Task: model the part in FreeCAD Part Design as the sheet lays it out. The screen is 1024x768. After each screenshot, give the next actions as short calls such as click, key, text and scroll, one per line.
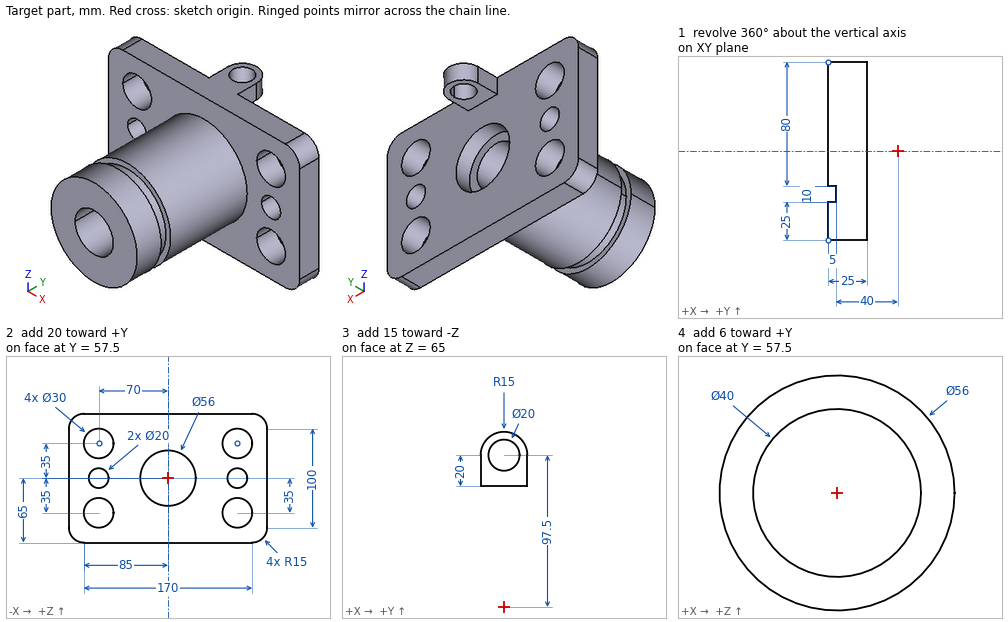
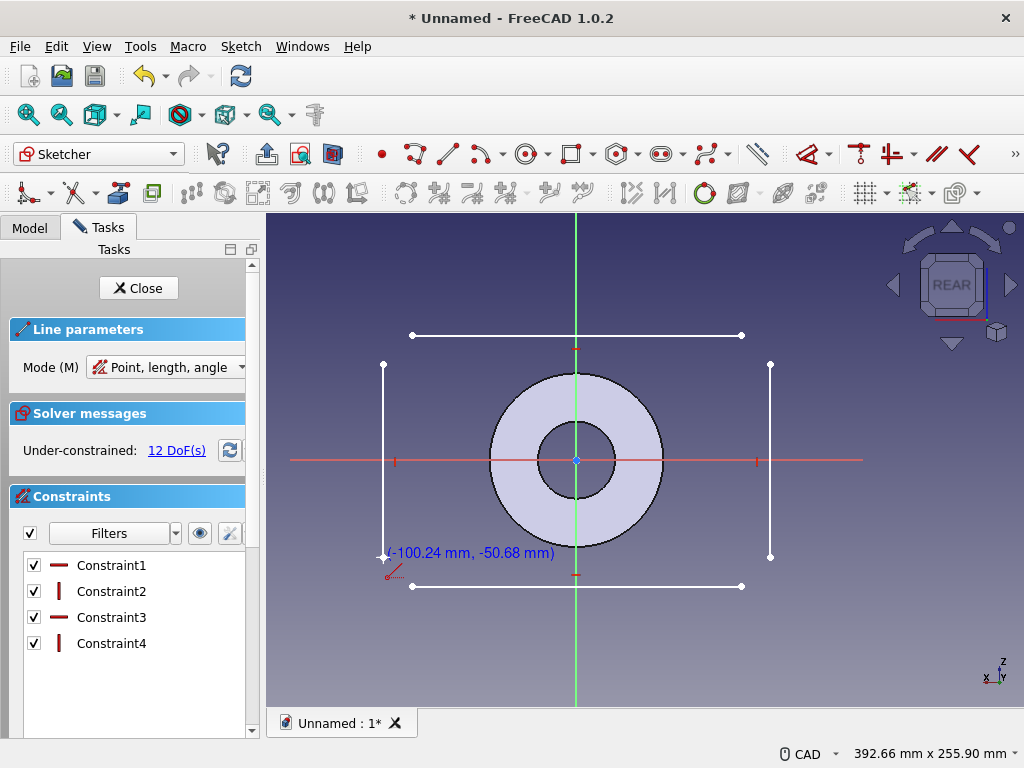
click(502, 154)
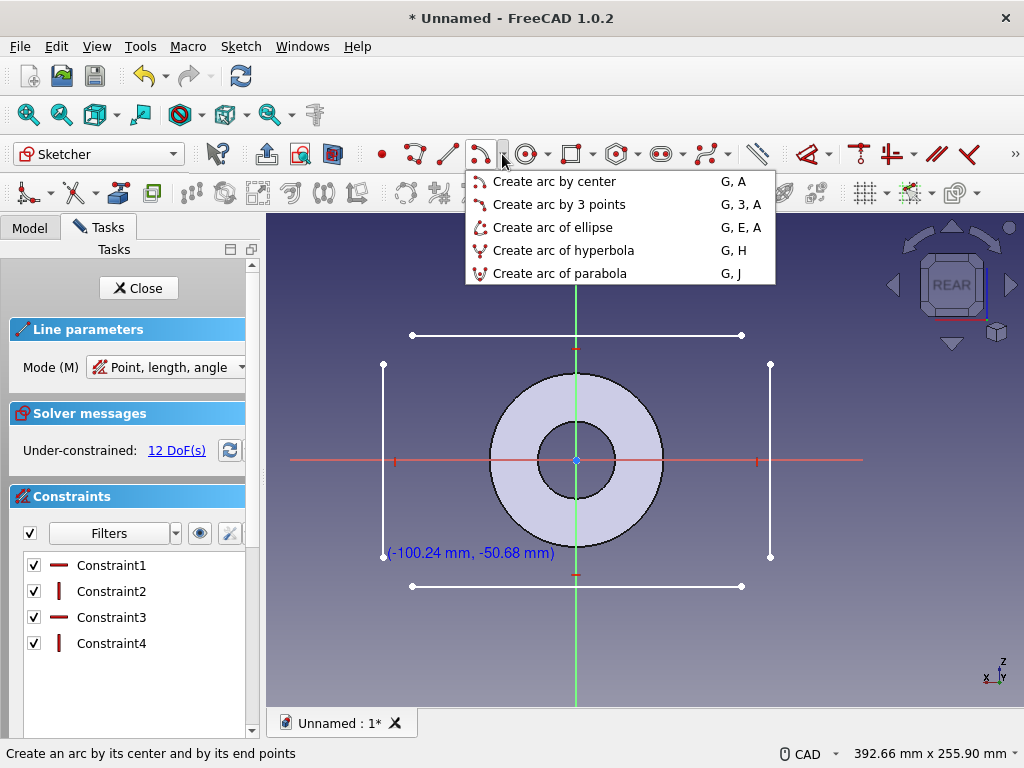
click(620, 204)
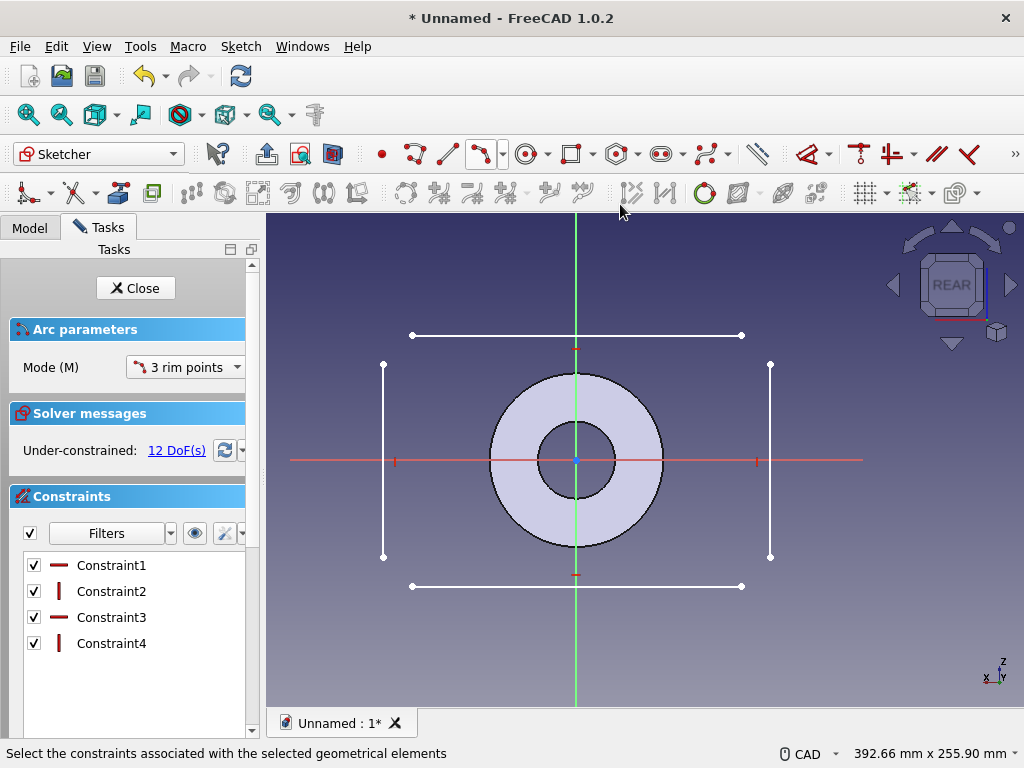
click(741, 587)
click(770, 558)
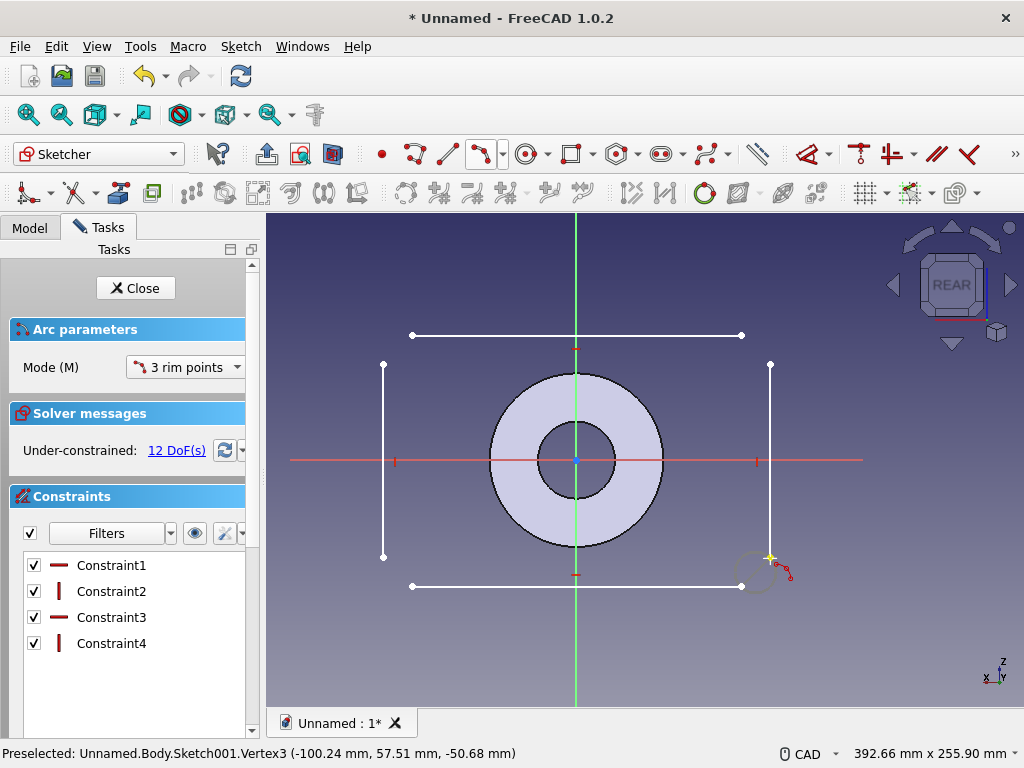
scroll(761, 577, up, 4)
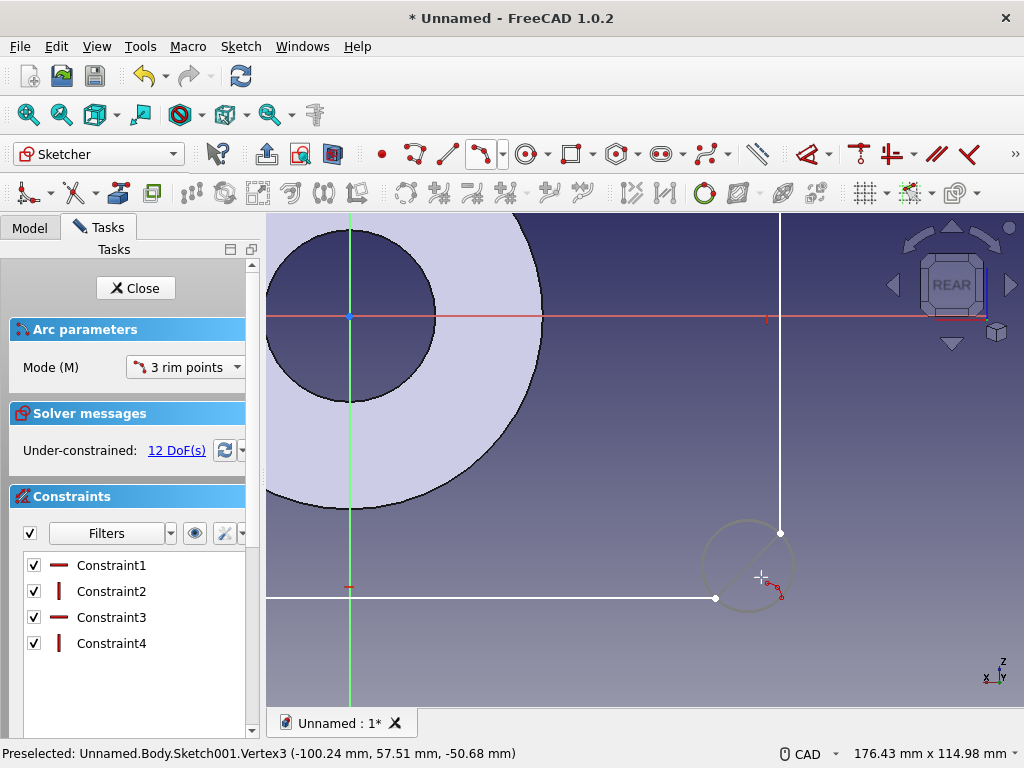
click(760, 576)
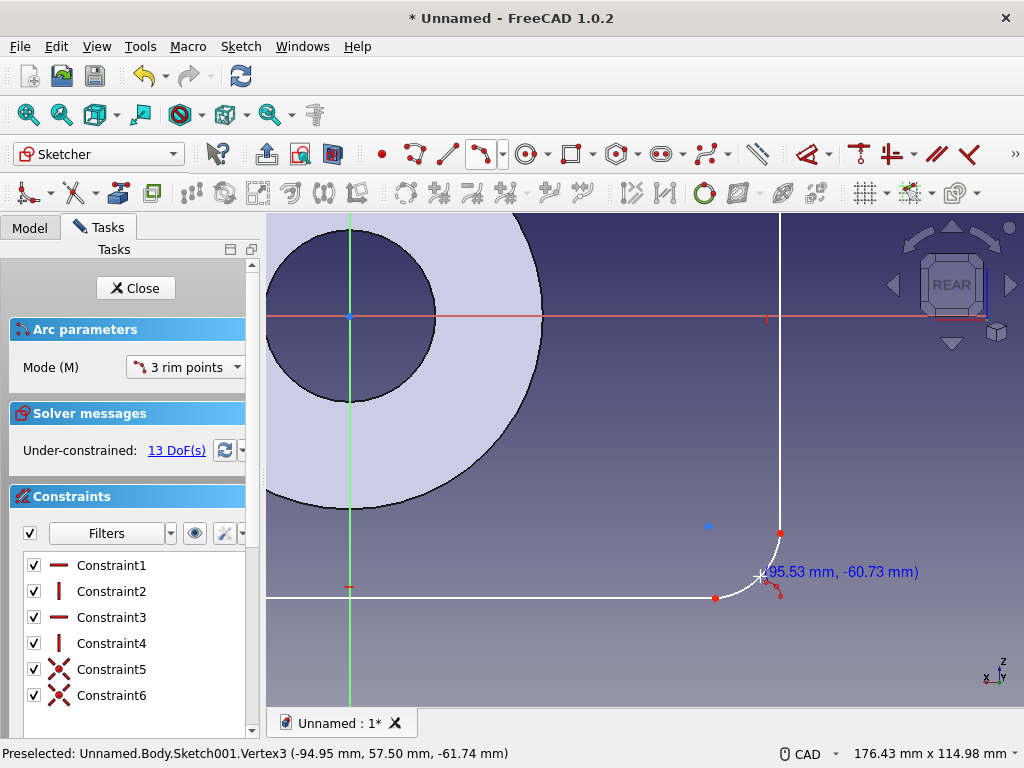
scroll(762, 577, down, 4)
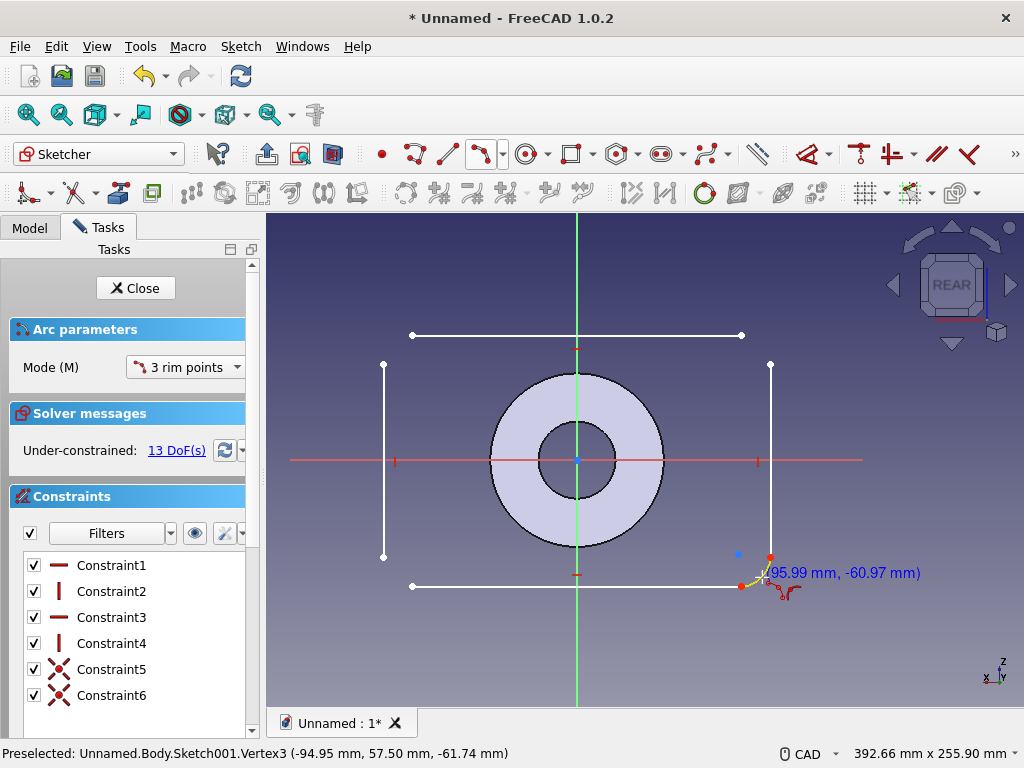
click(771, 365)
click(742, 336)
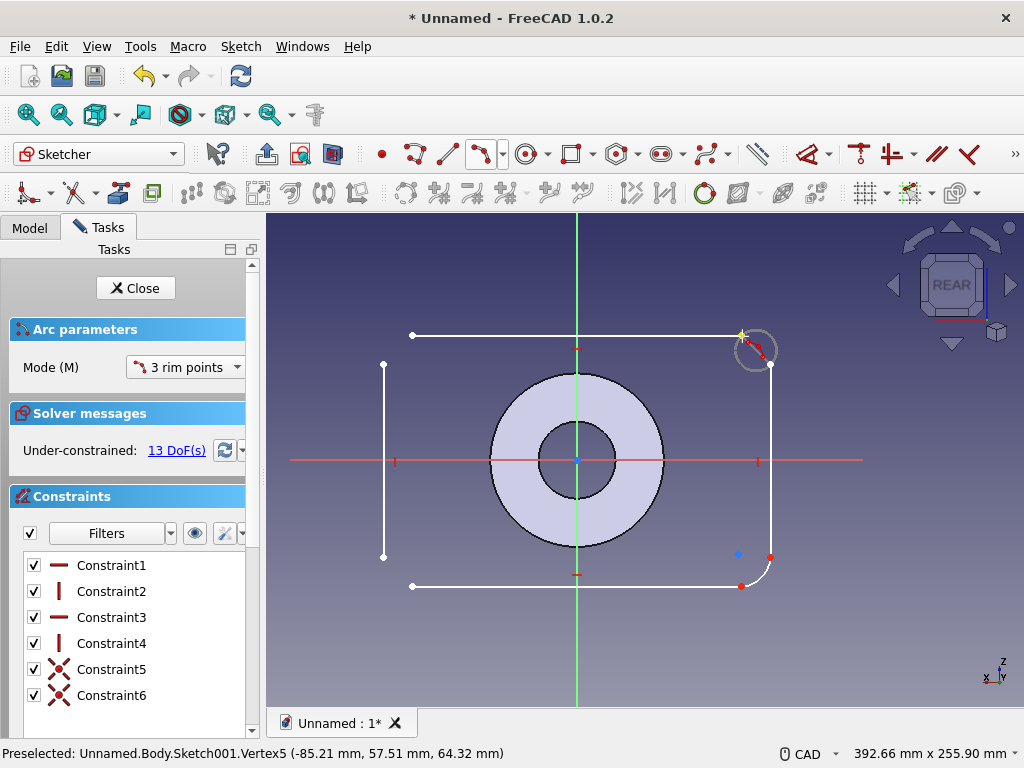
scroll(762, 343, up, 4)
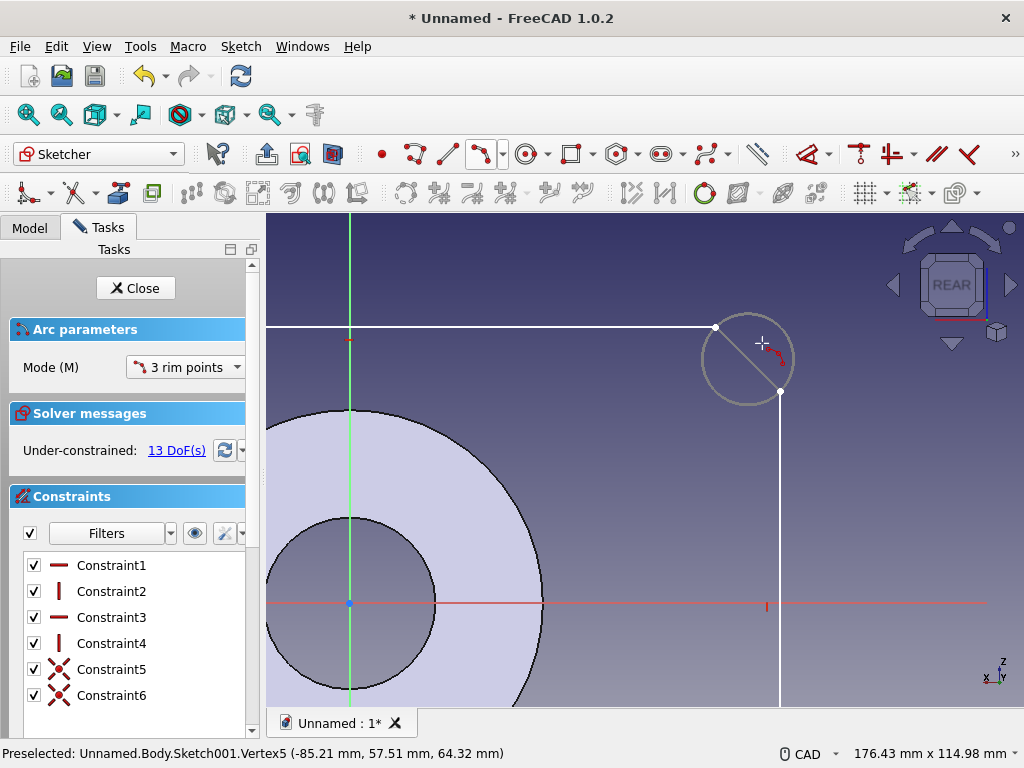
click(760, 343)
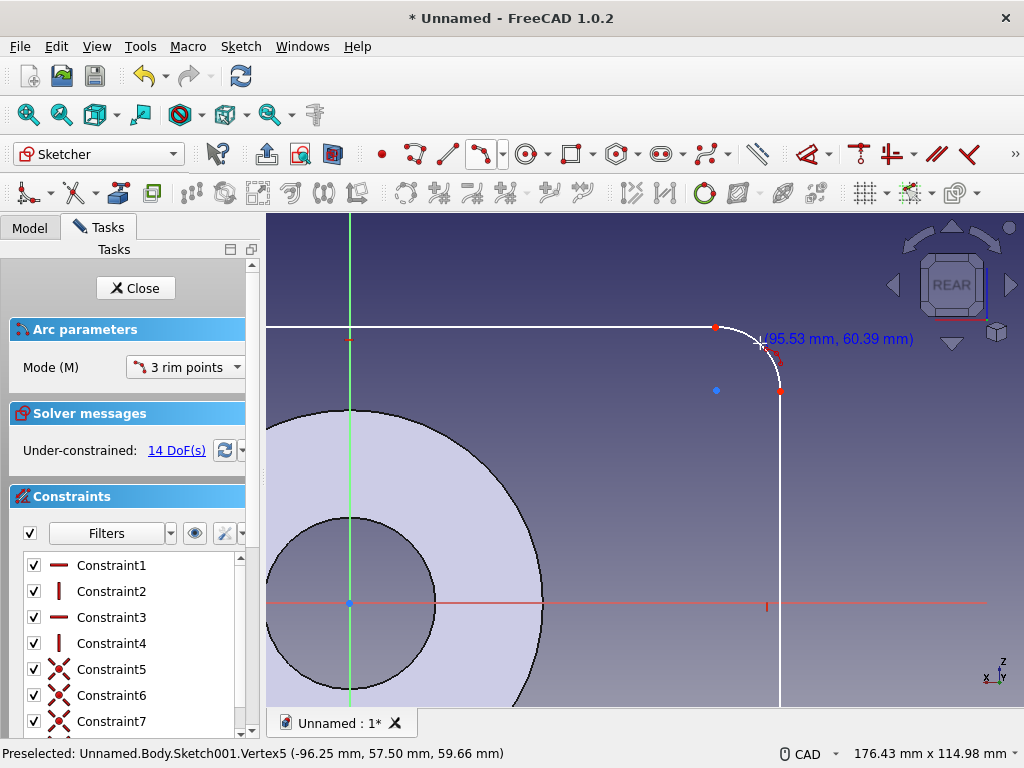
scroll(762, 343, down, 4)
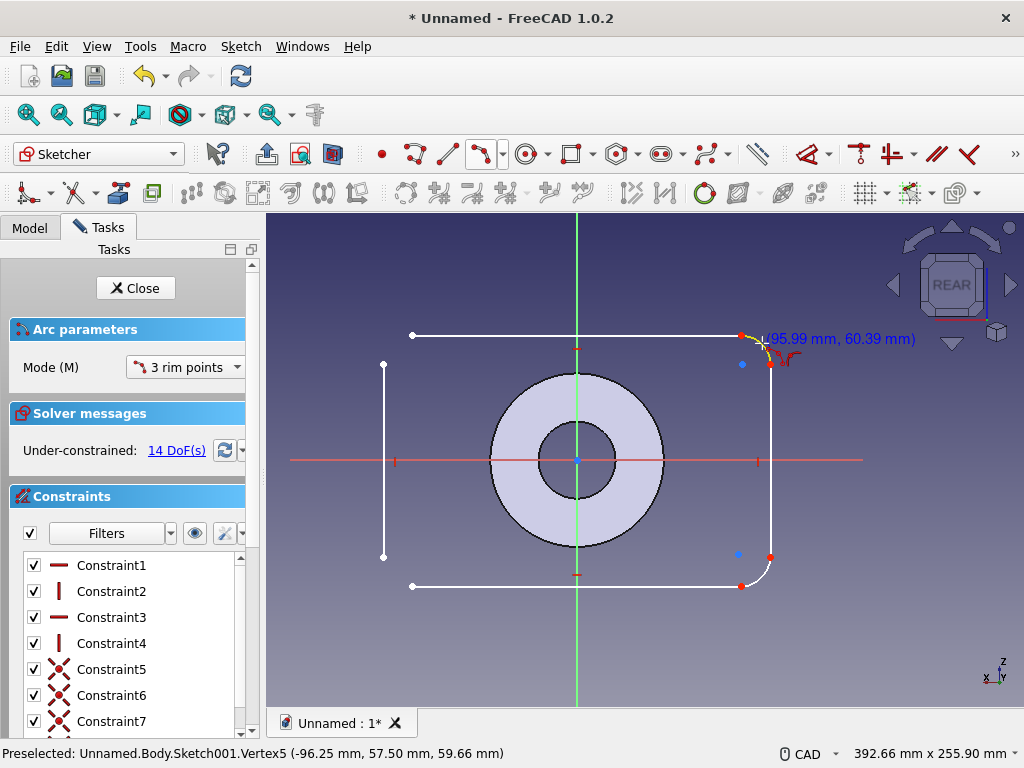
click(413, 336)
click(384, 365)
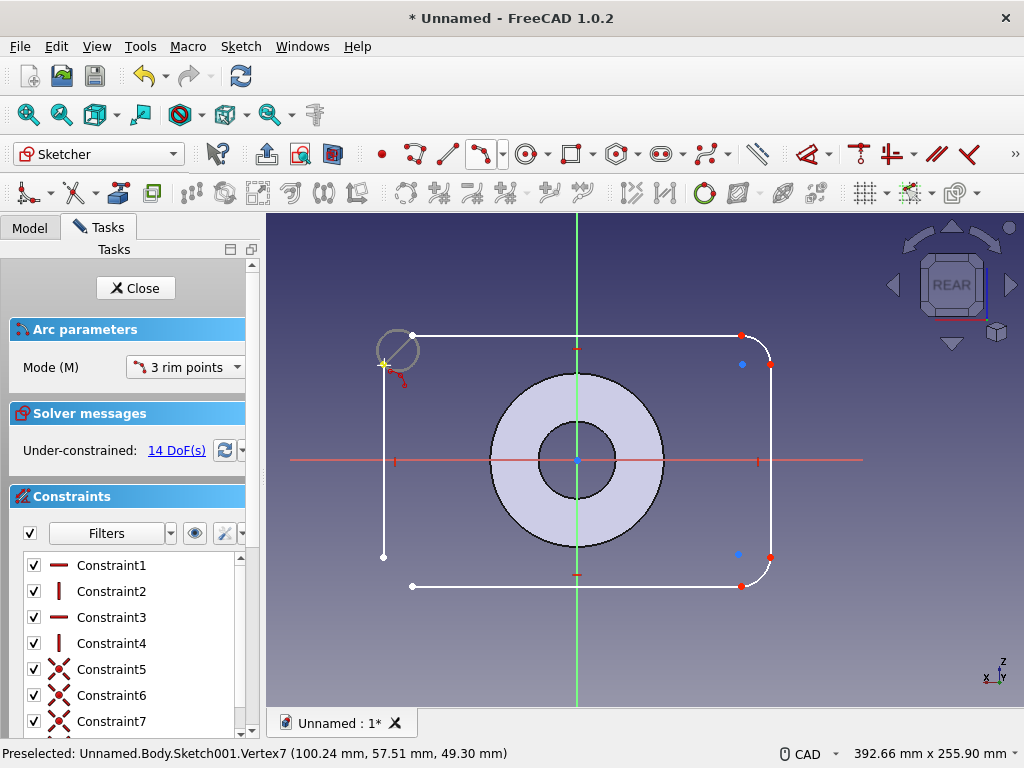
scroll(392, 343, up, 4)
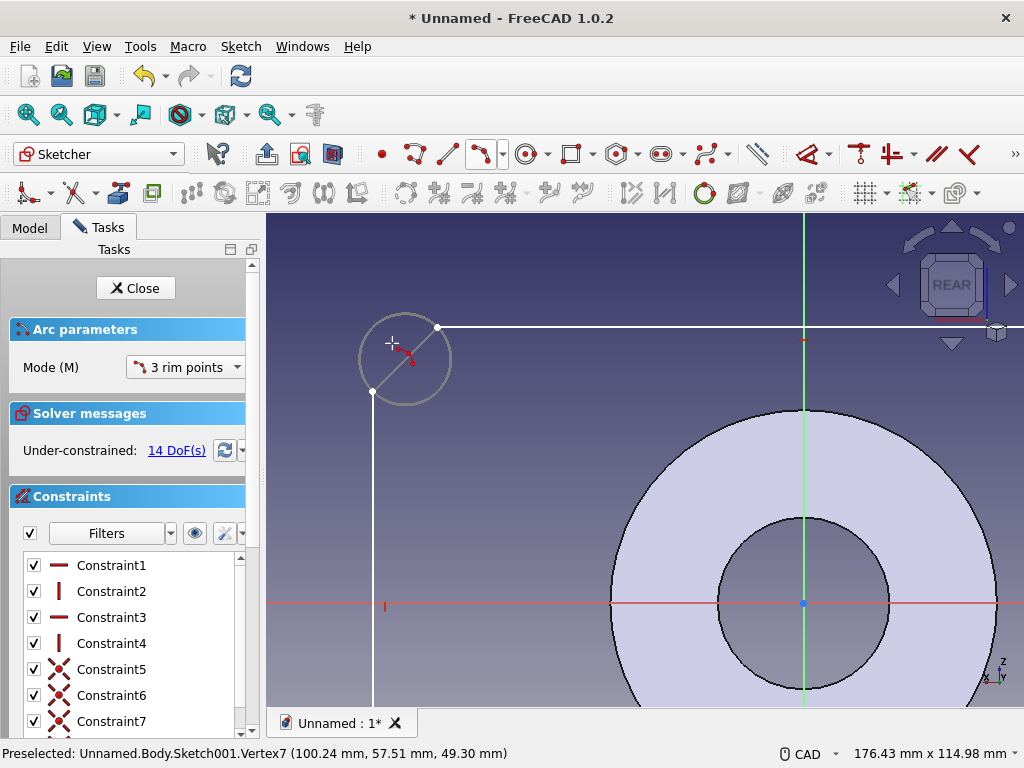
click(393, 343)